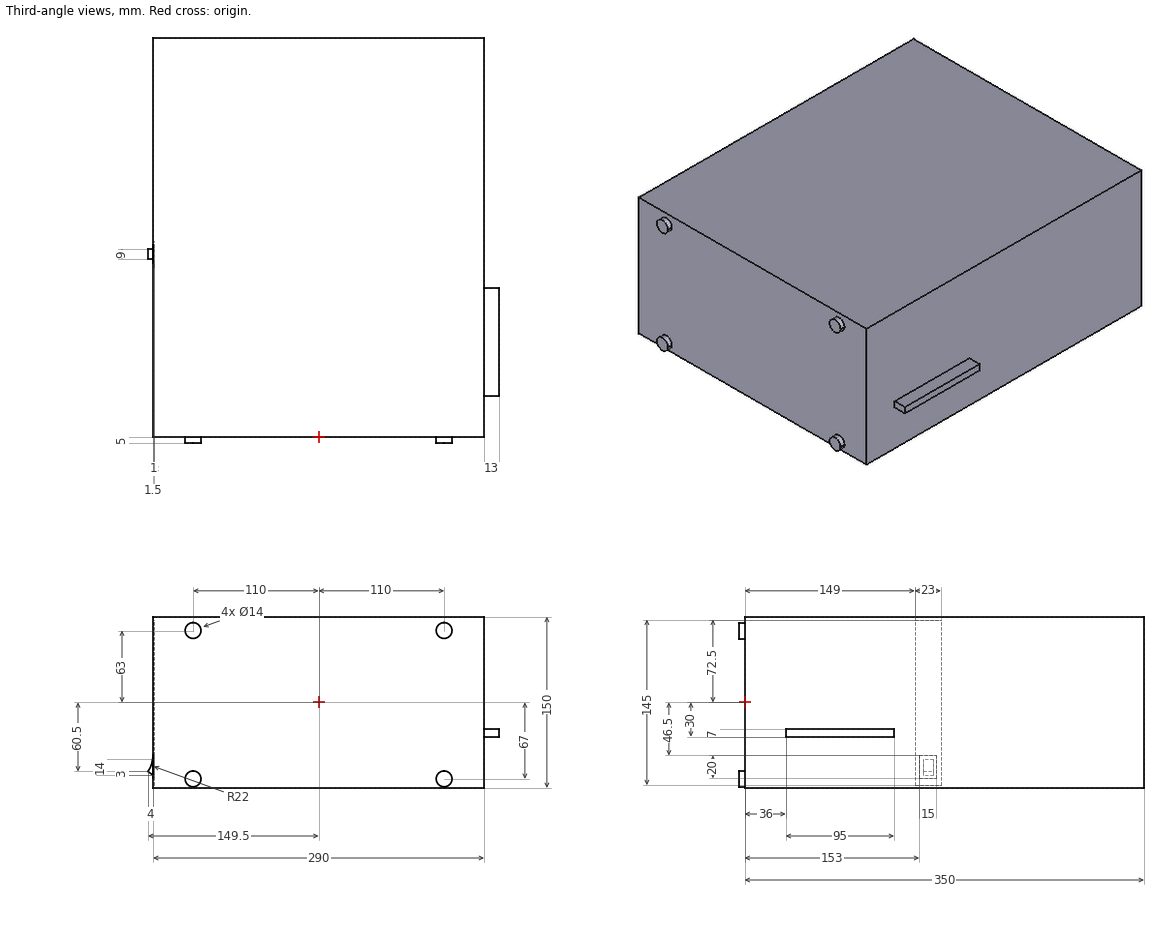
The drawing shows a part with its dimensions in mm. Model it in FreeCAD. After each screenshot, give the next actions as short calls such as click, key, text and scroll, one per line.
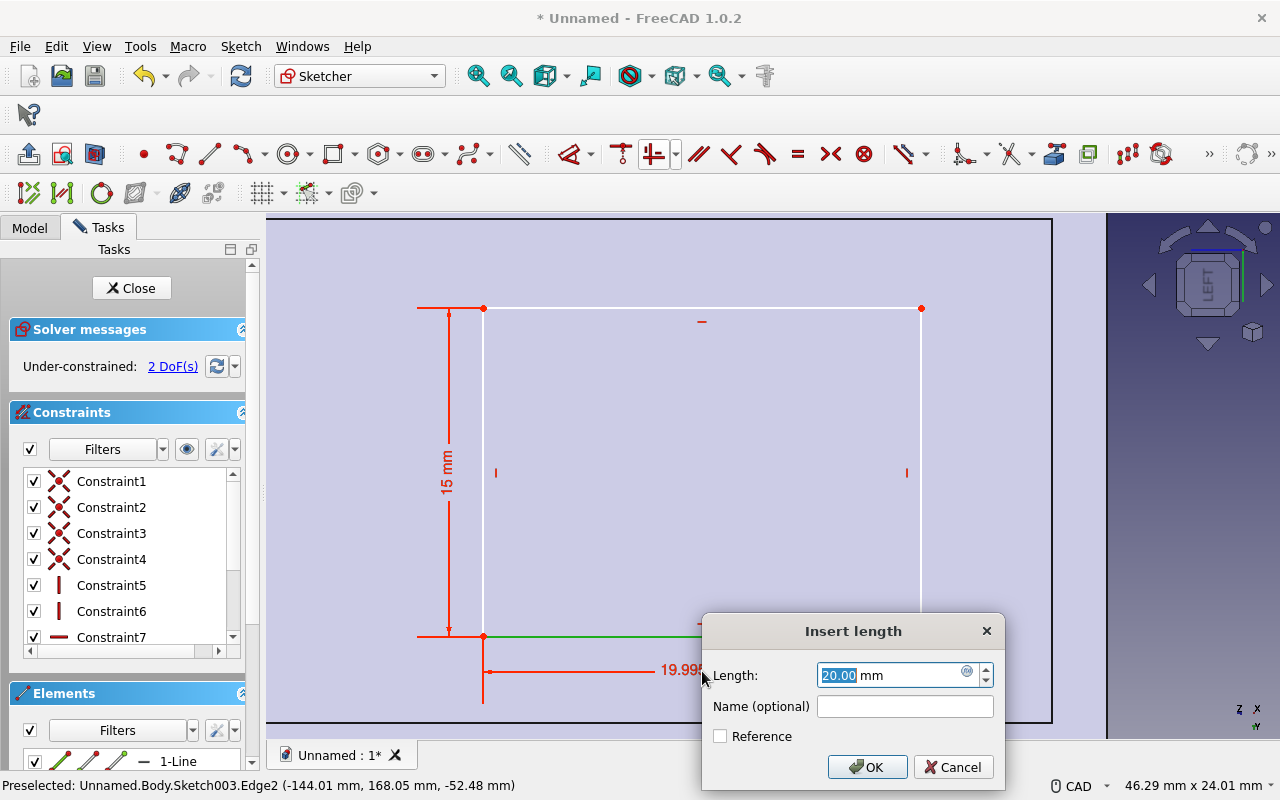
text(20)
key(Return)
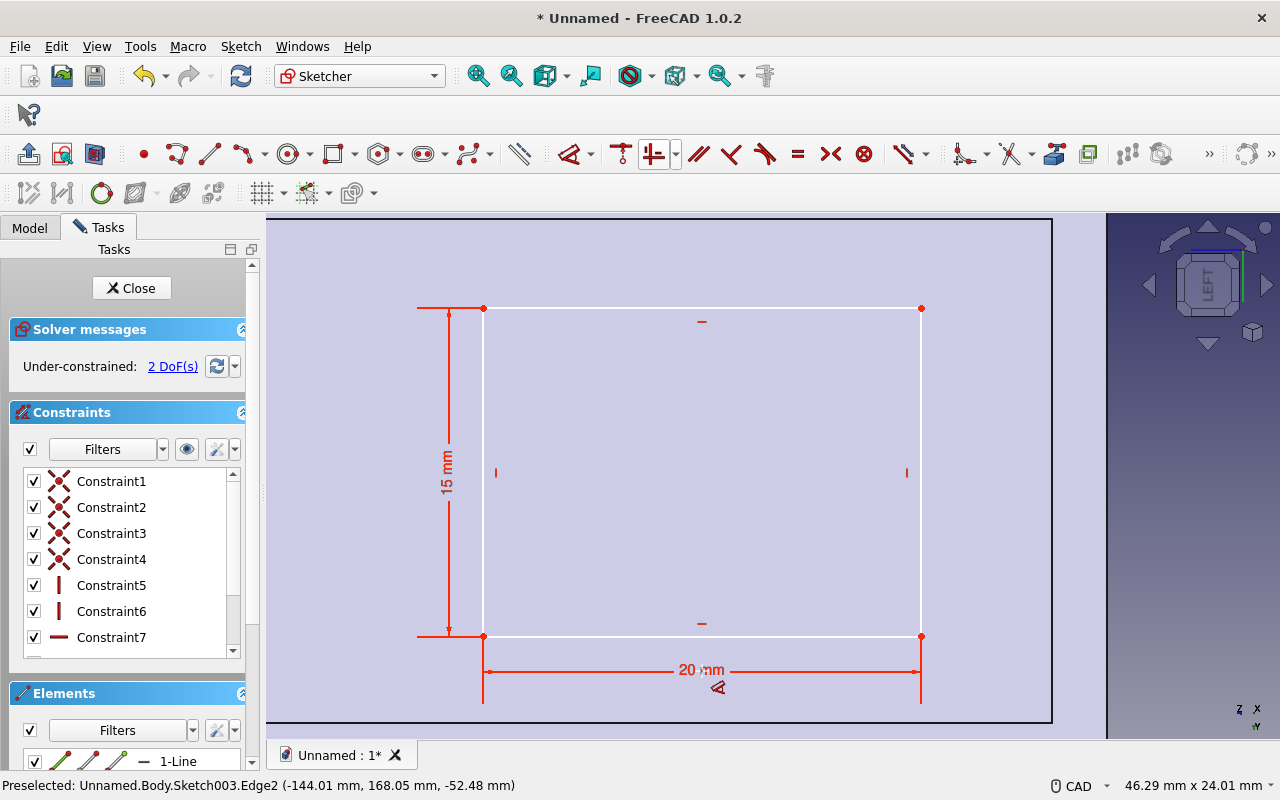
click(483, 308)
click(517, 275)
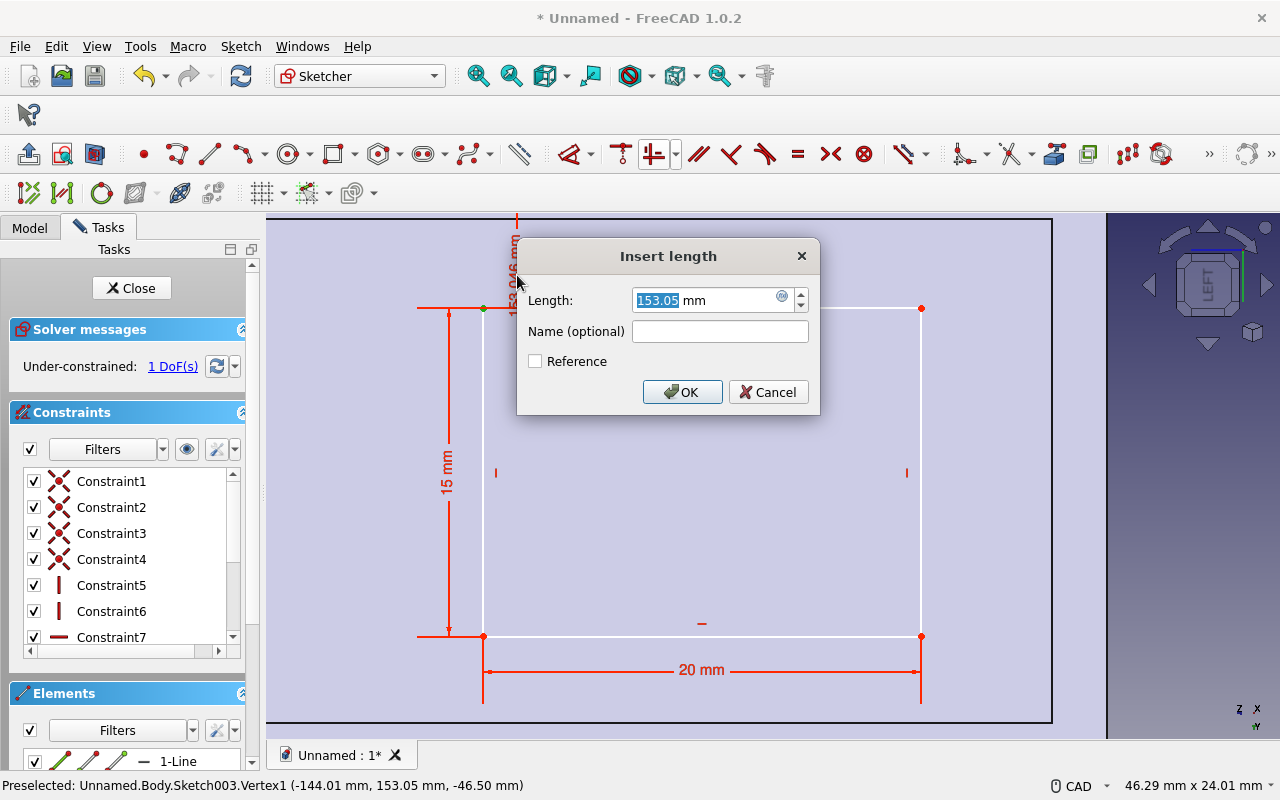
text(153)
key(Return)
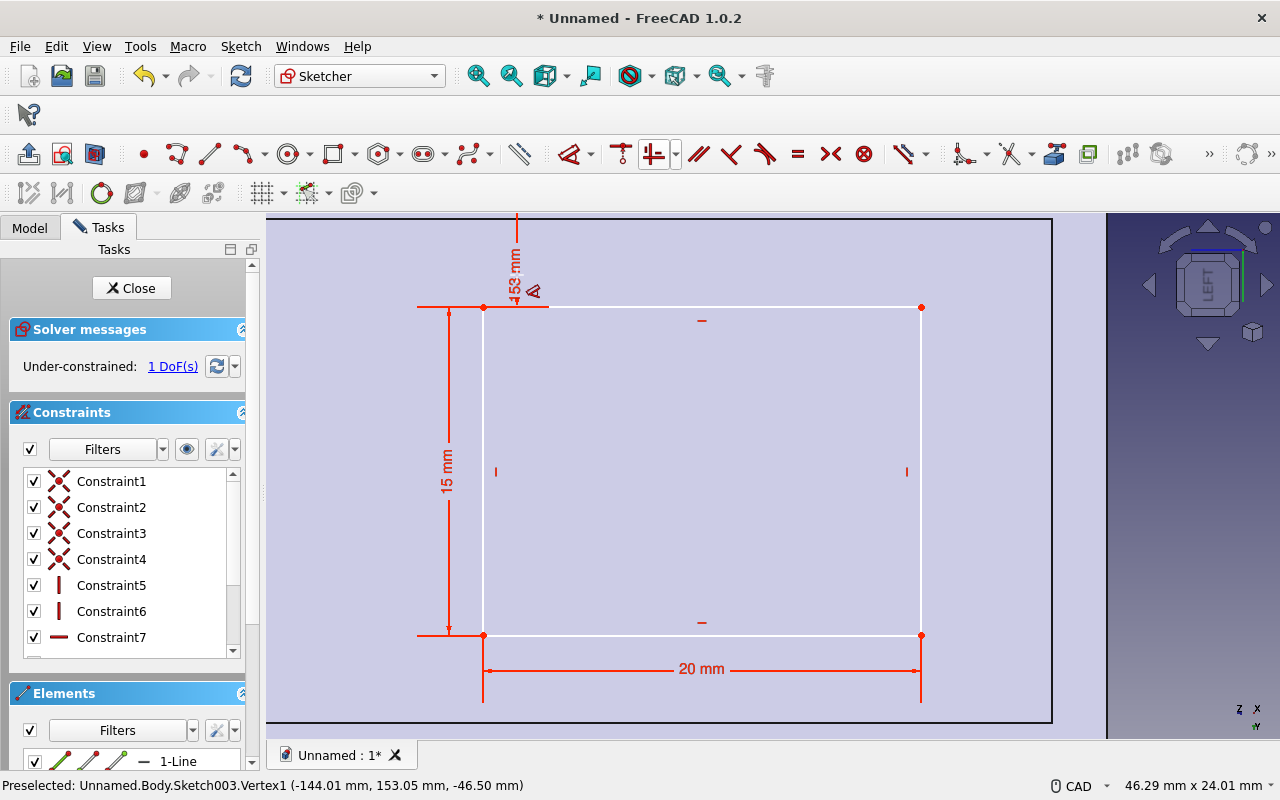
click(483, 307)
click(388, 341)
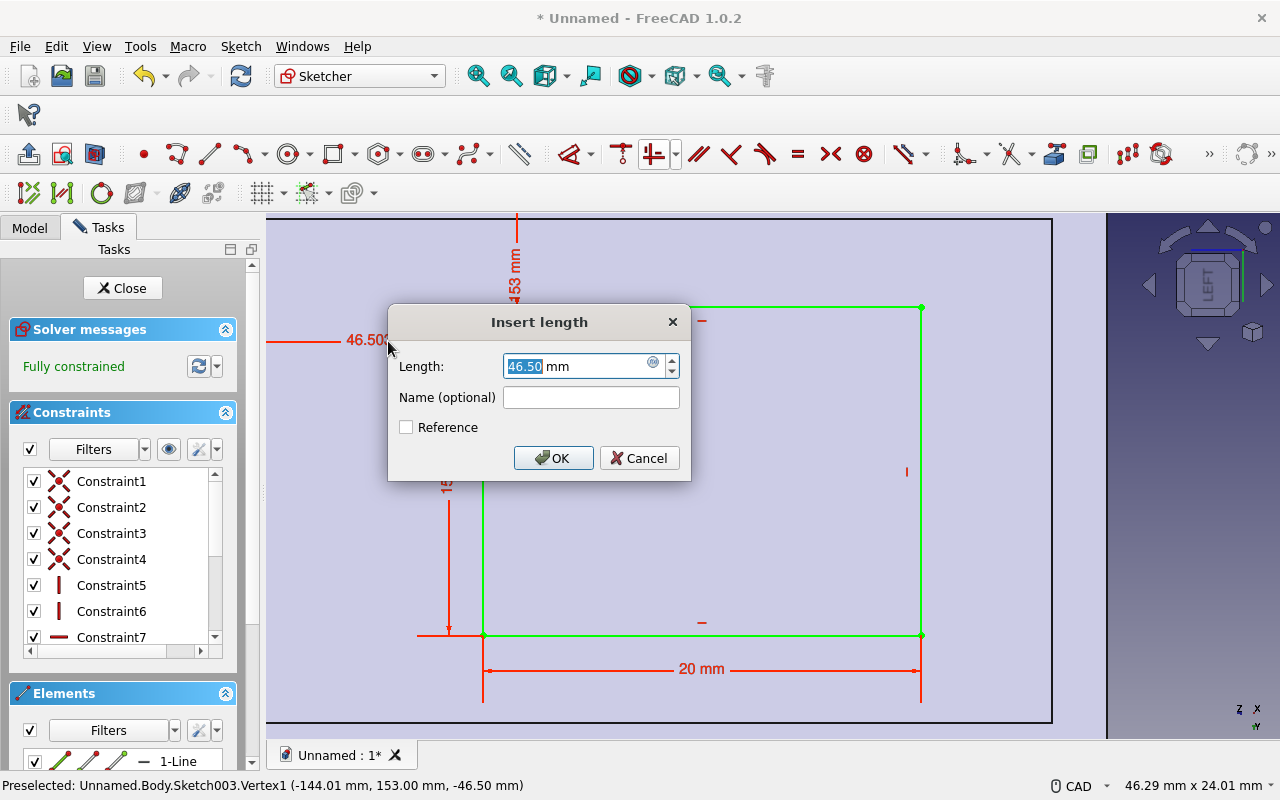
text(46.5)
key(Return)
key(Escape)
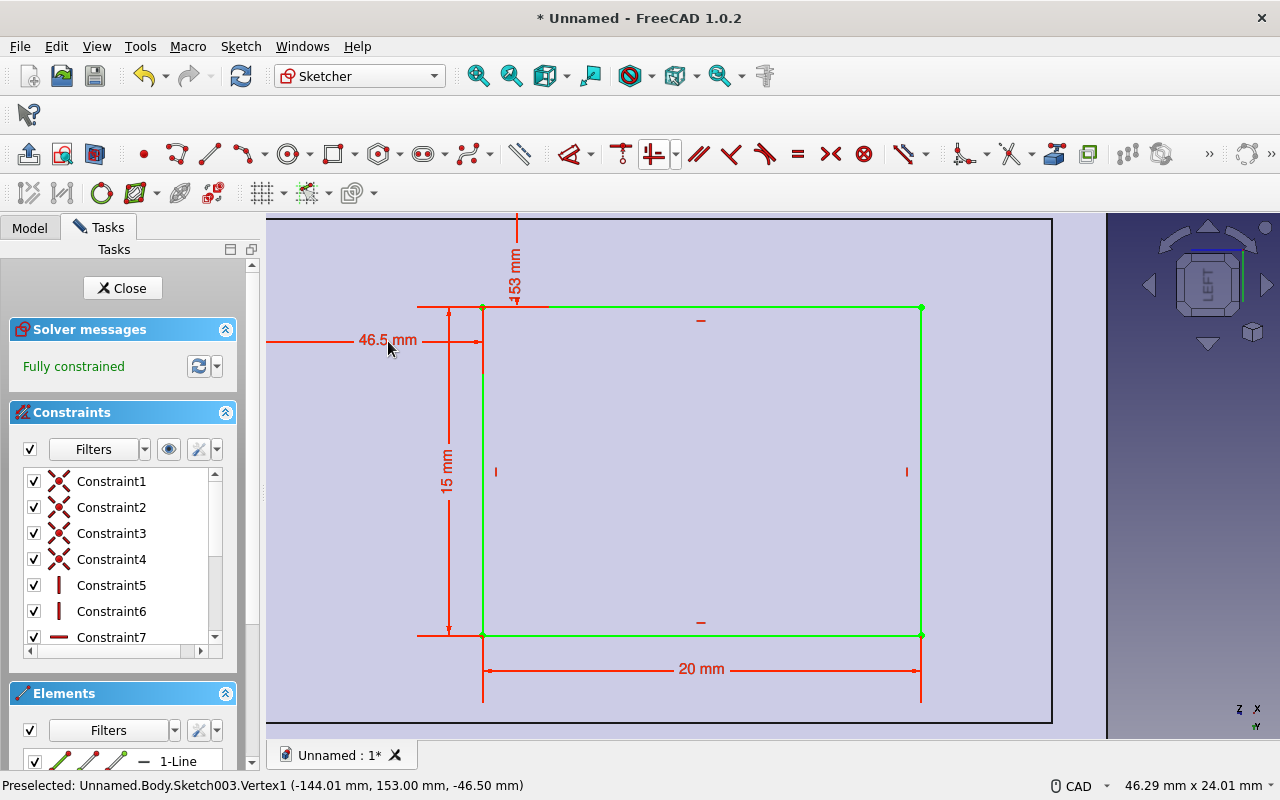
click(123, 288)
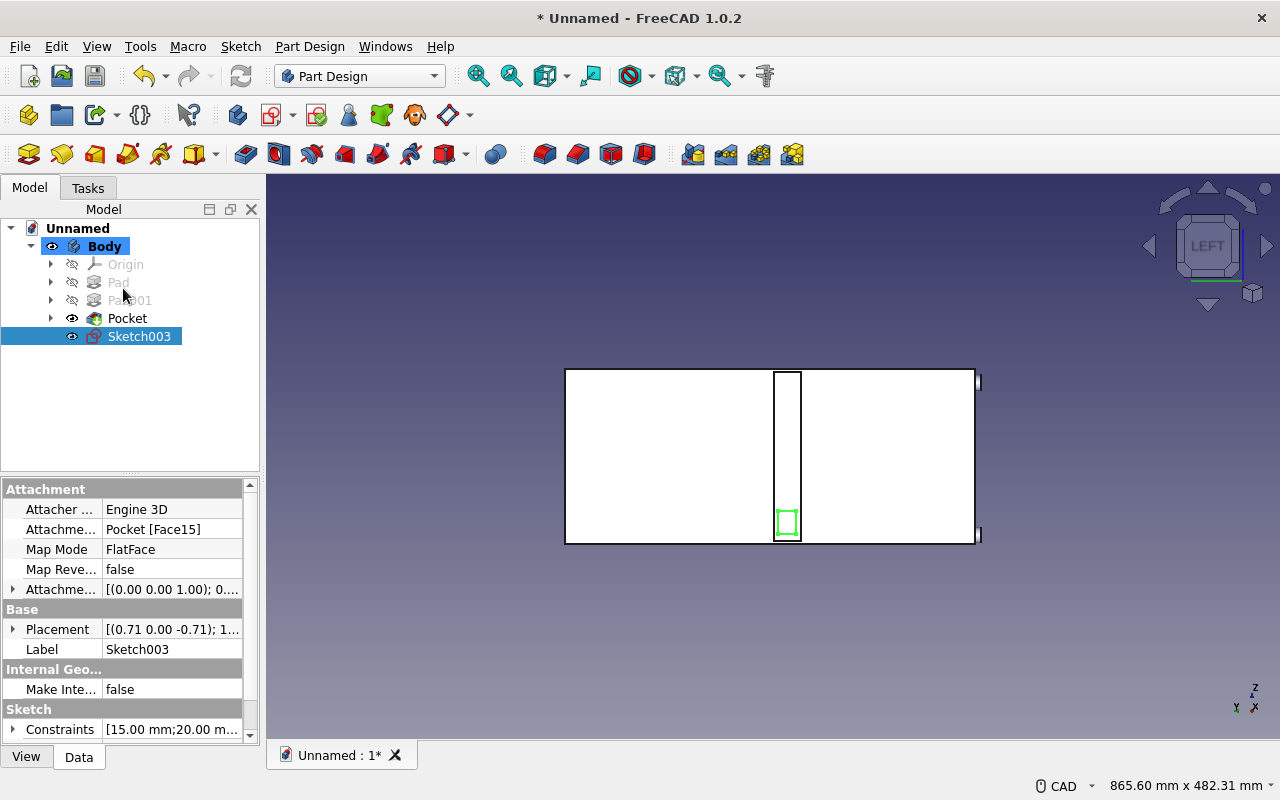
click(29, 154)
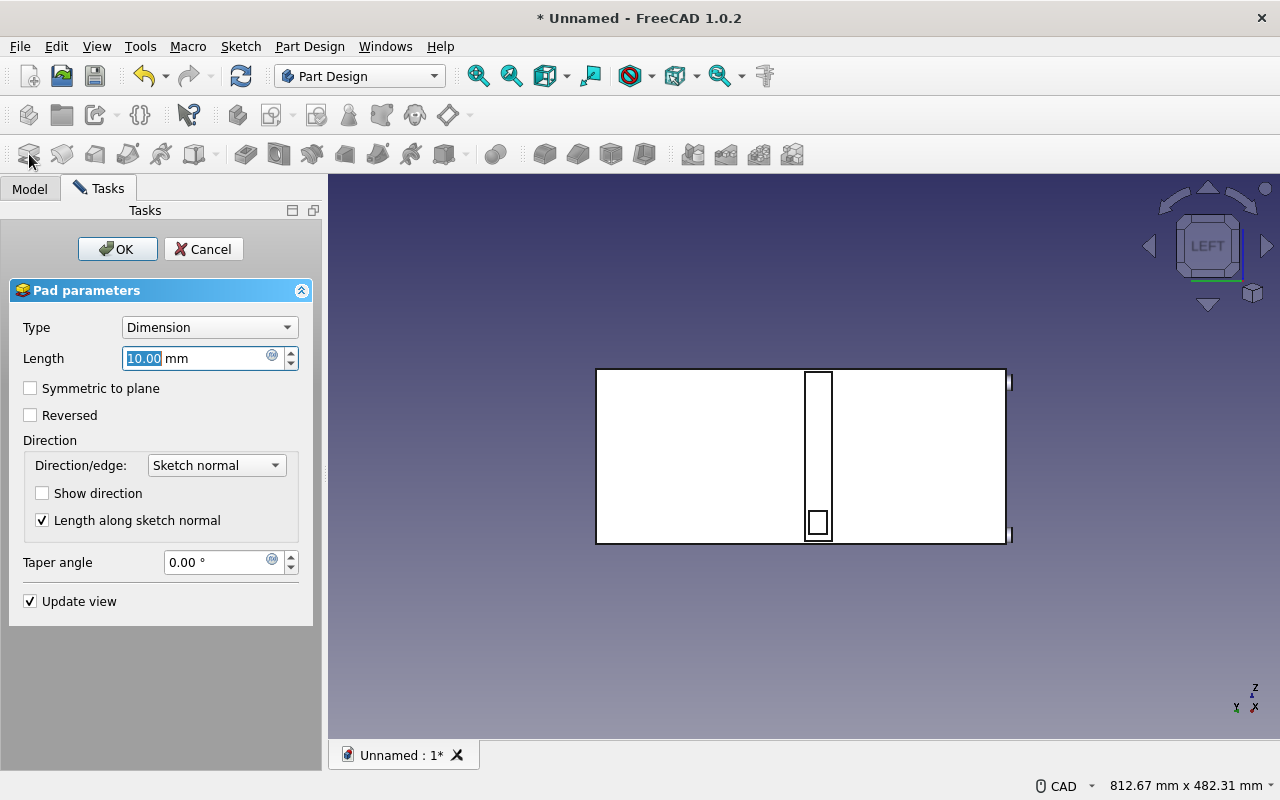
text(1.5)
key(Tab)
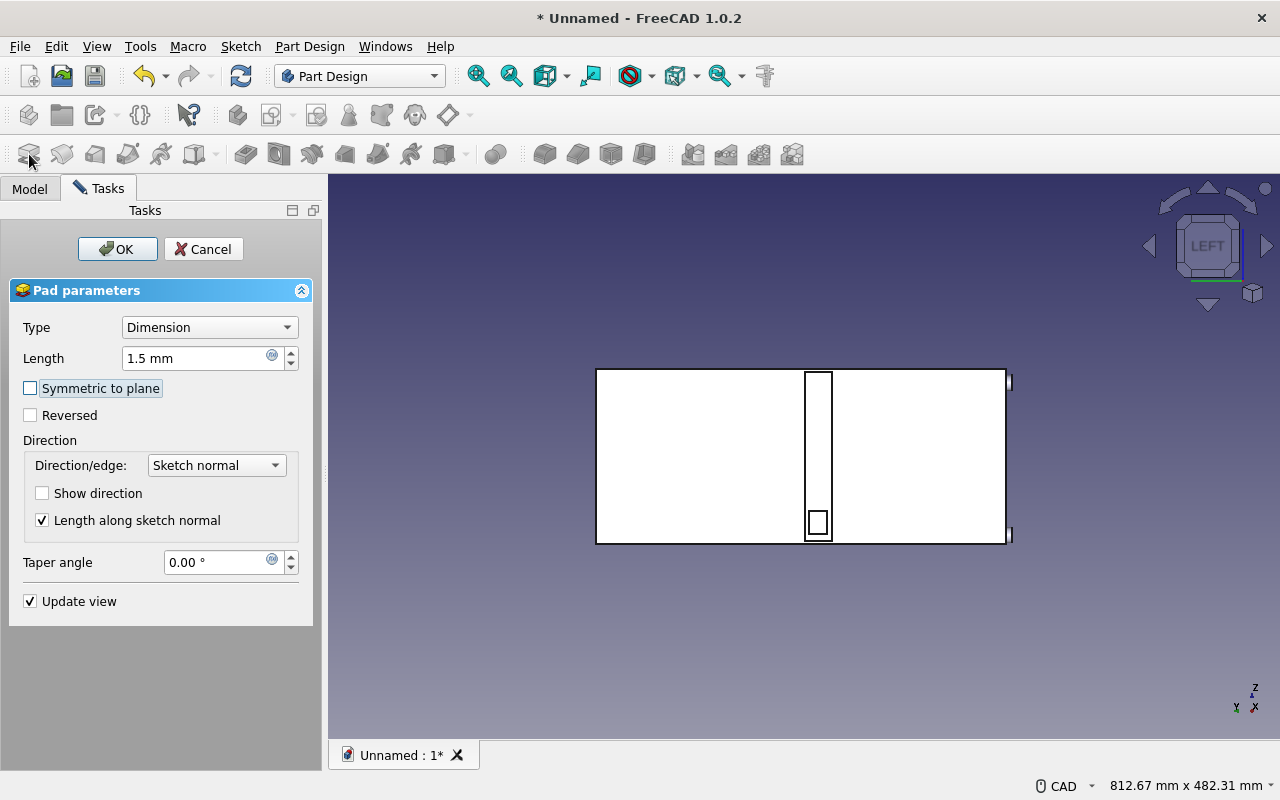
click(118, 249)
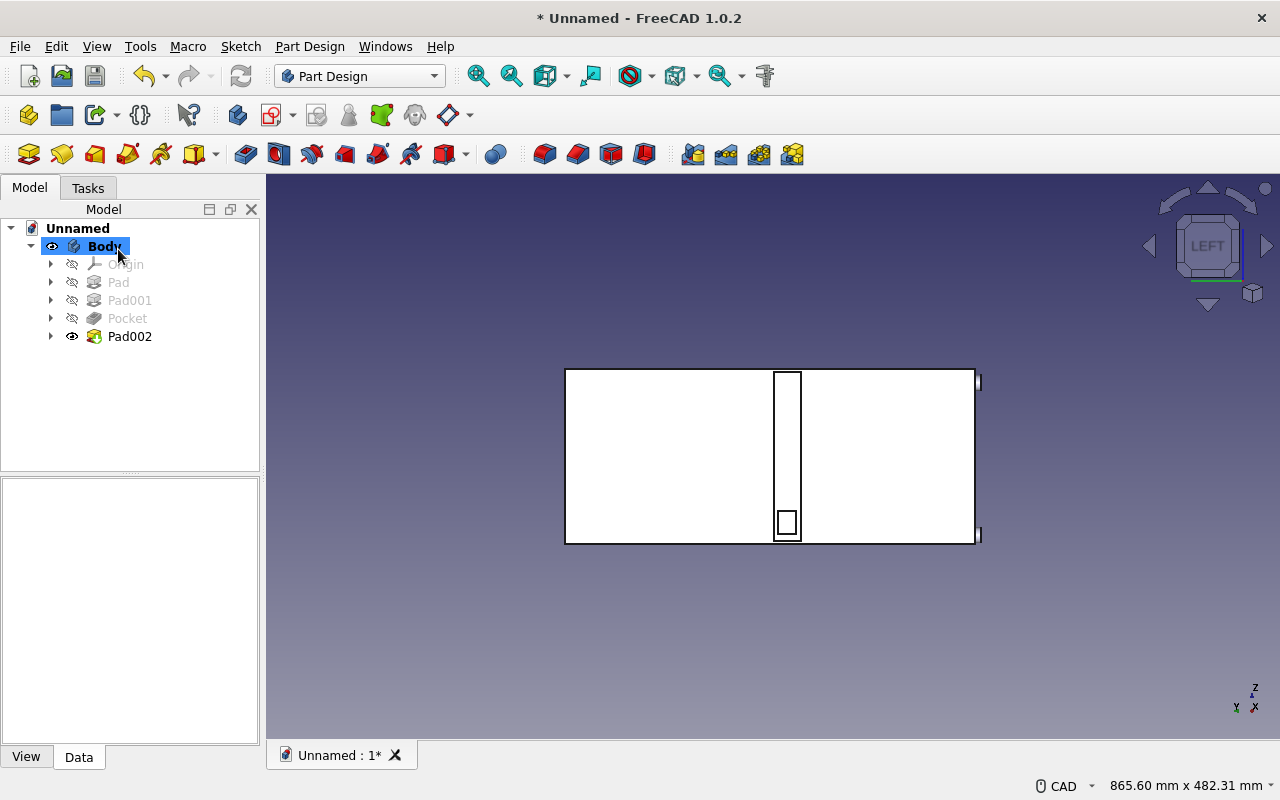
click(479, 76)